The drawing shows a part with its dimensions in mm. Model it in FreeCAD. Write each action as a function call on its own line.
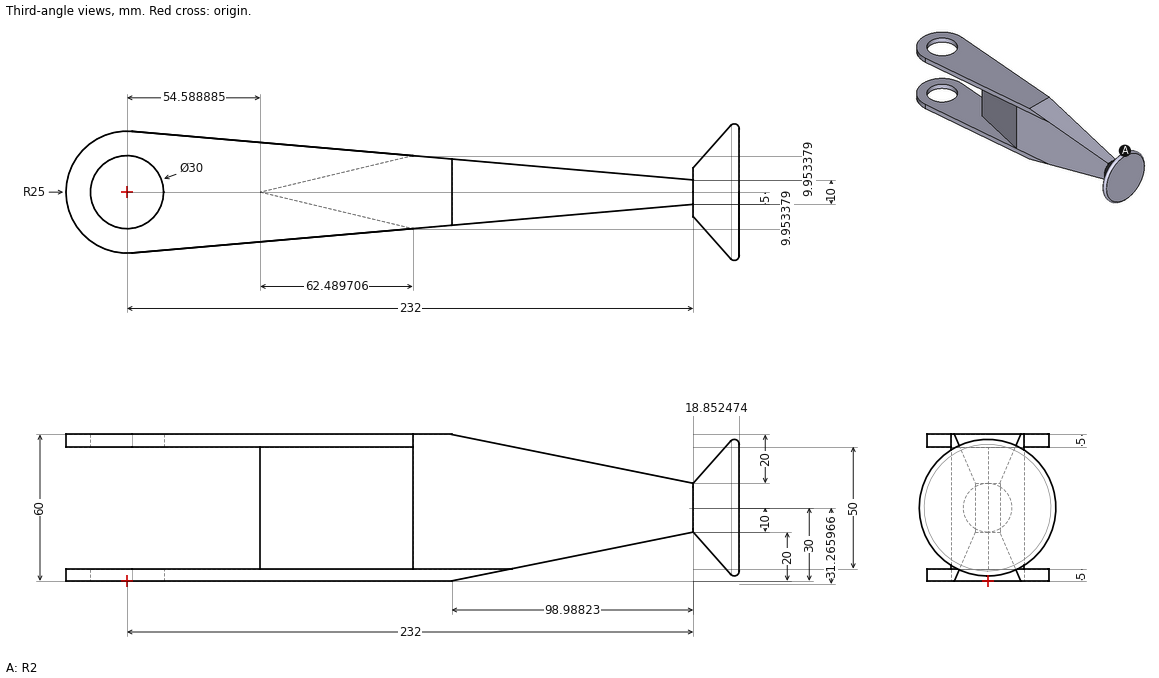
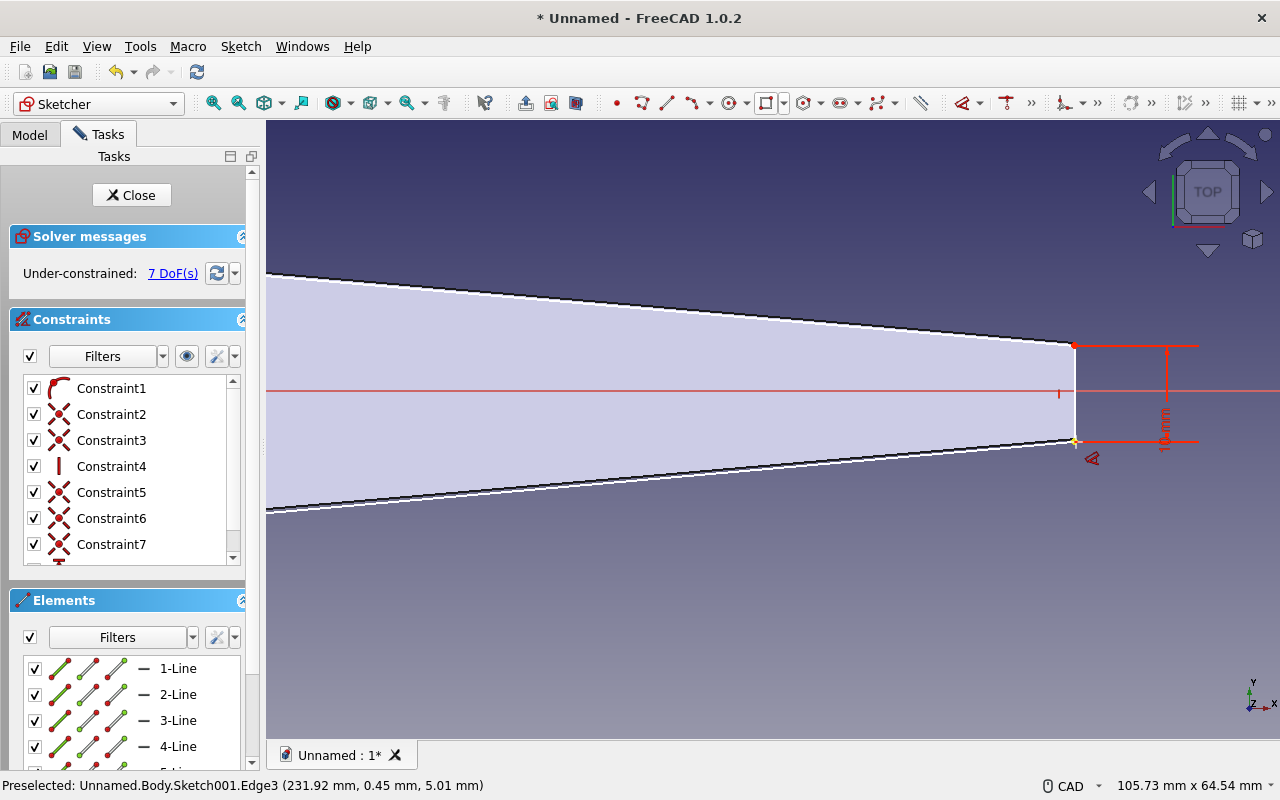
click(1075, 442)
click(1109, 405)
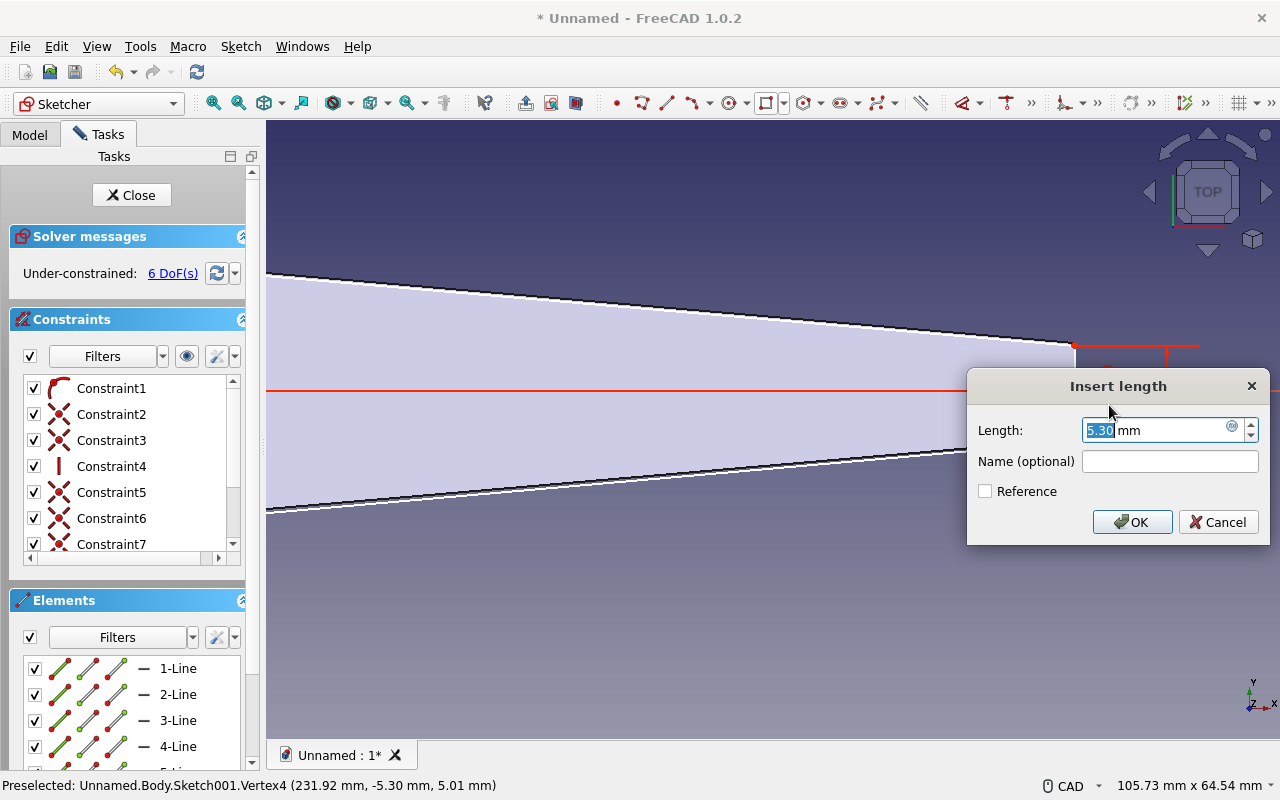
text(5)
key(Return)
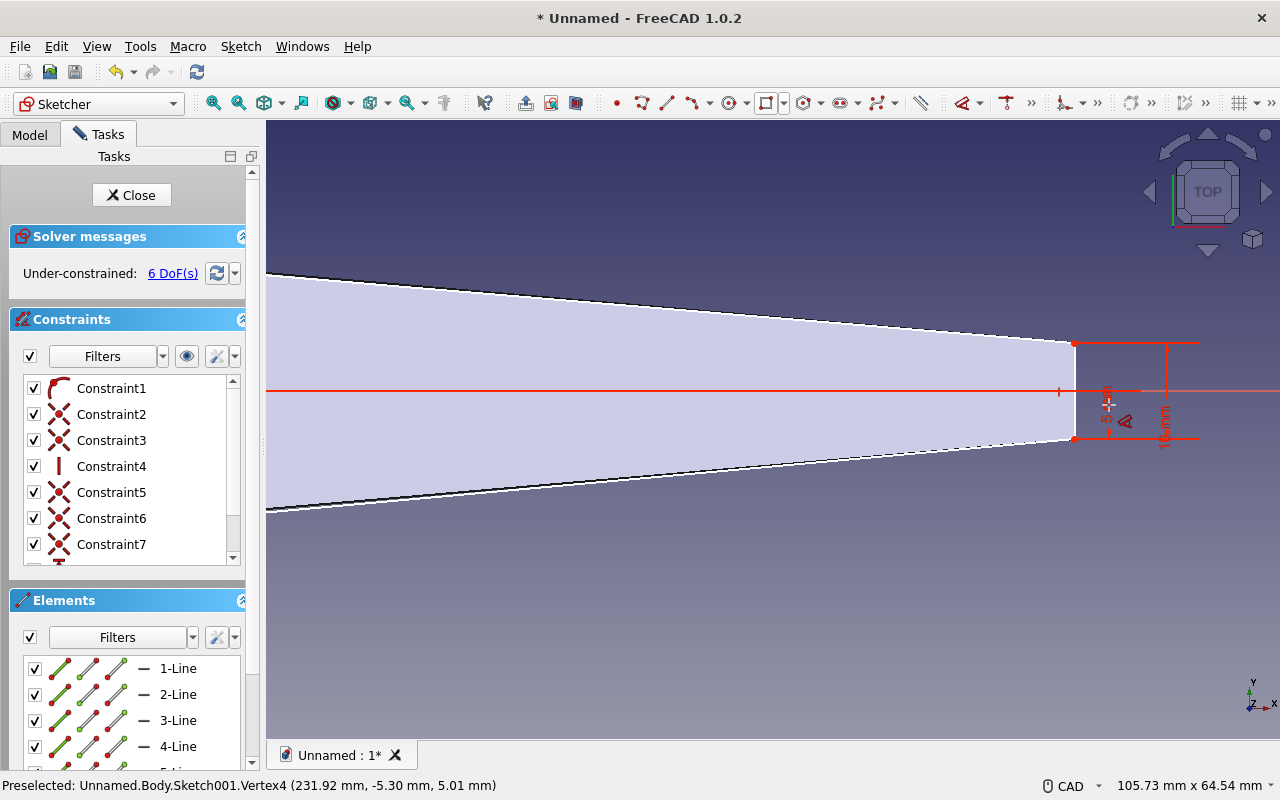
scroll(947, 442, down, 7)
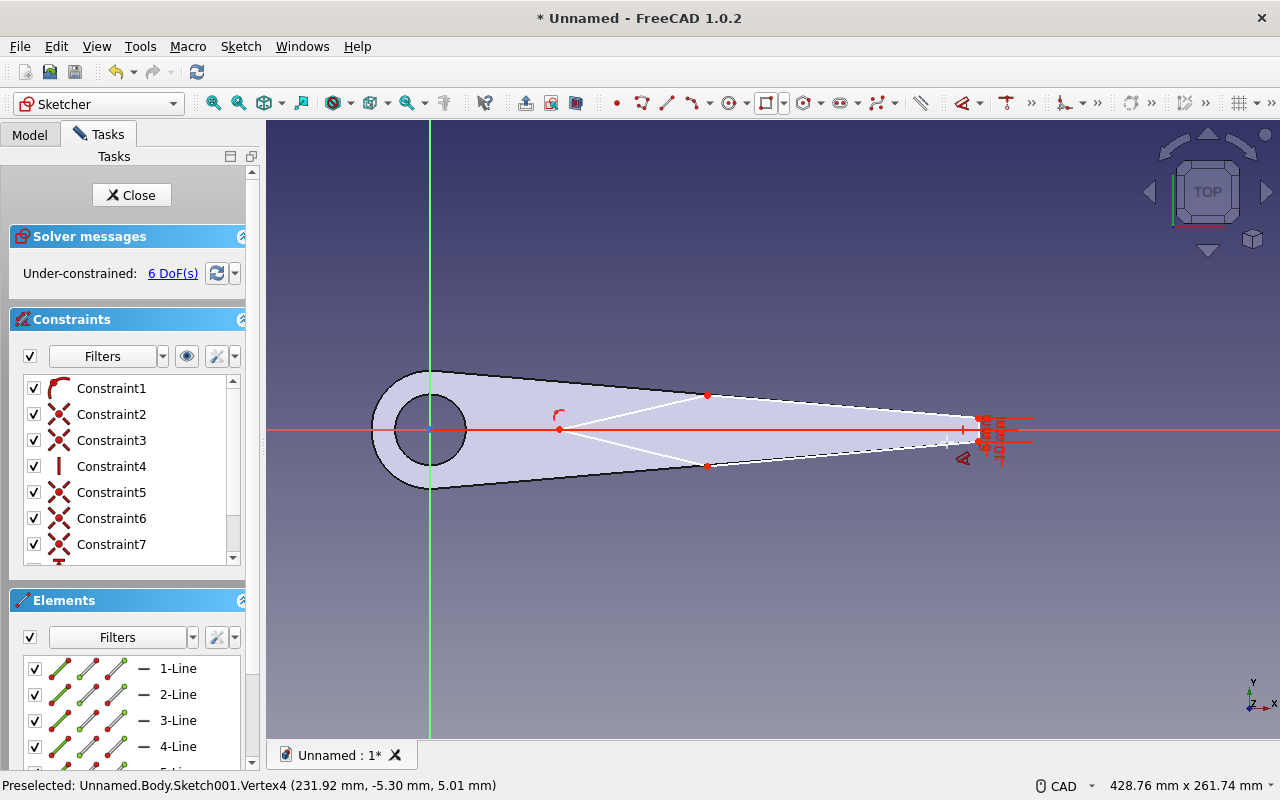
click(979, 442)
click(579, 476)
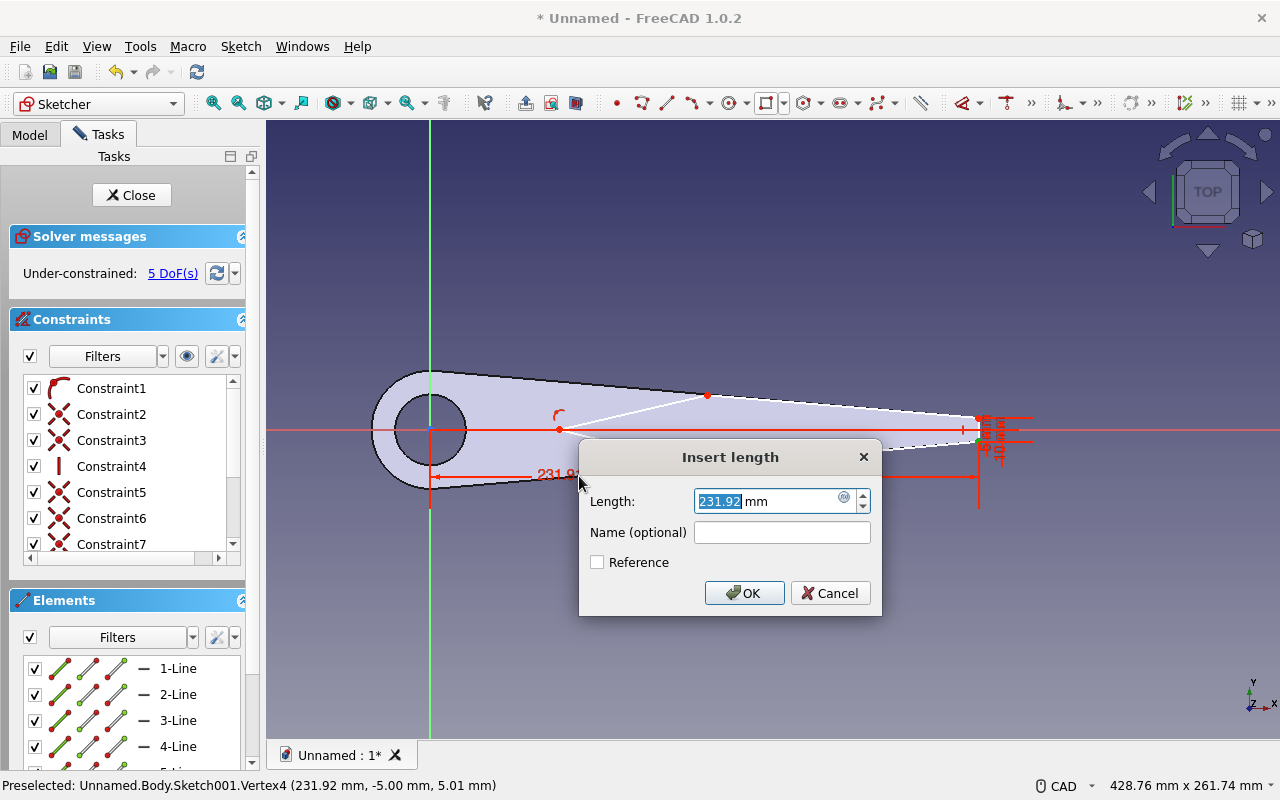
text(232)
key(Return)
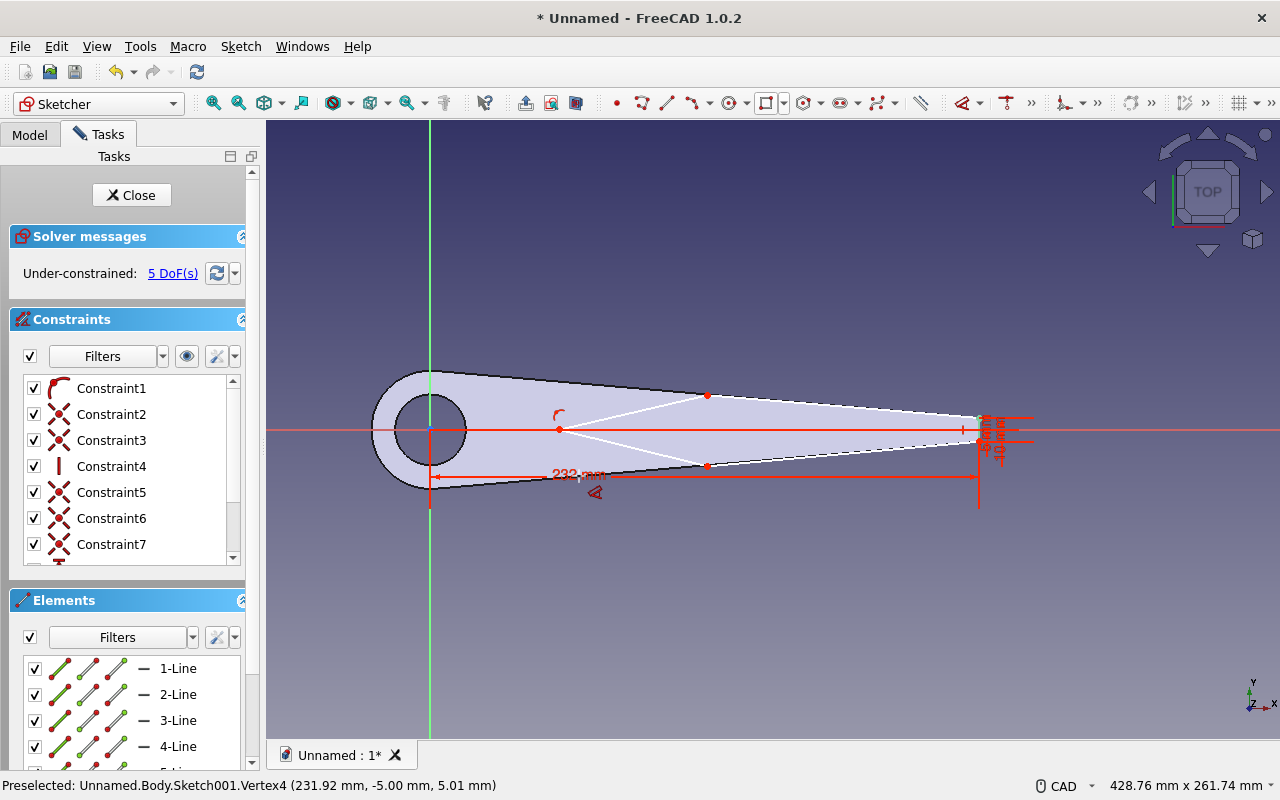
scroll(789, 459, up, 3)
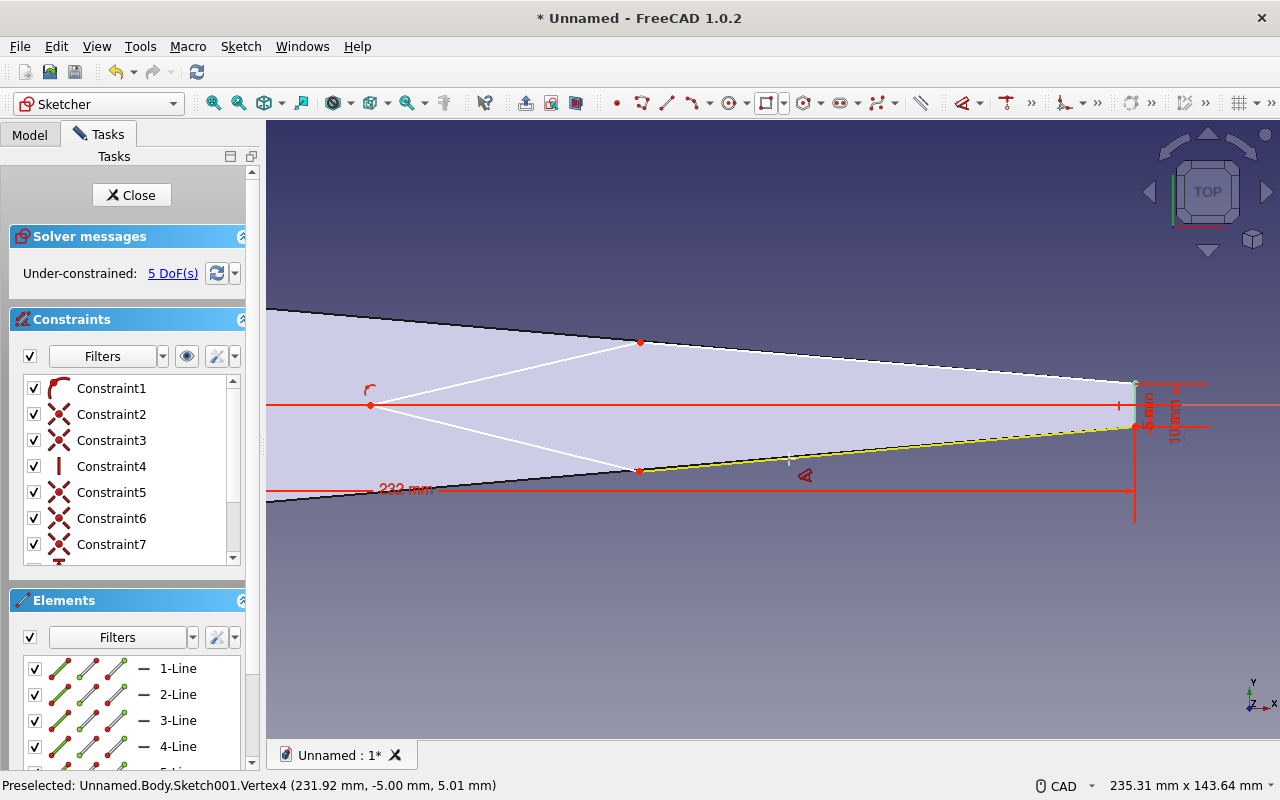
click(788, 458)
click(606, 449)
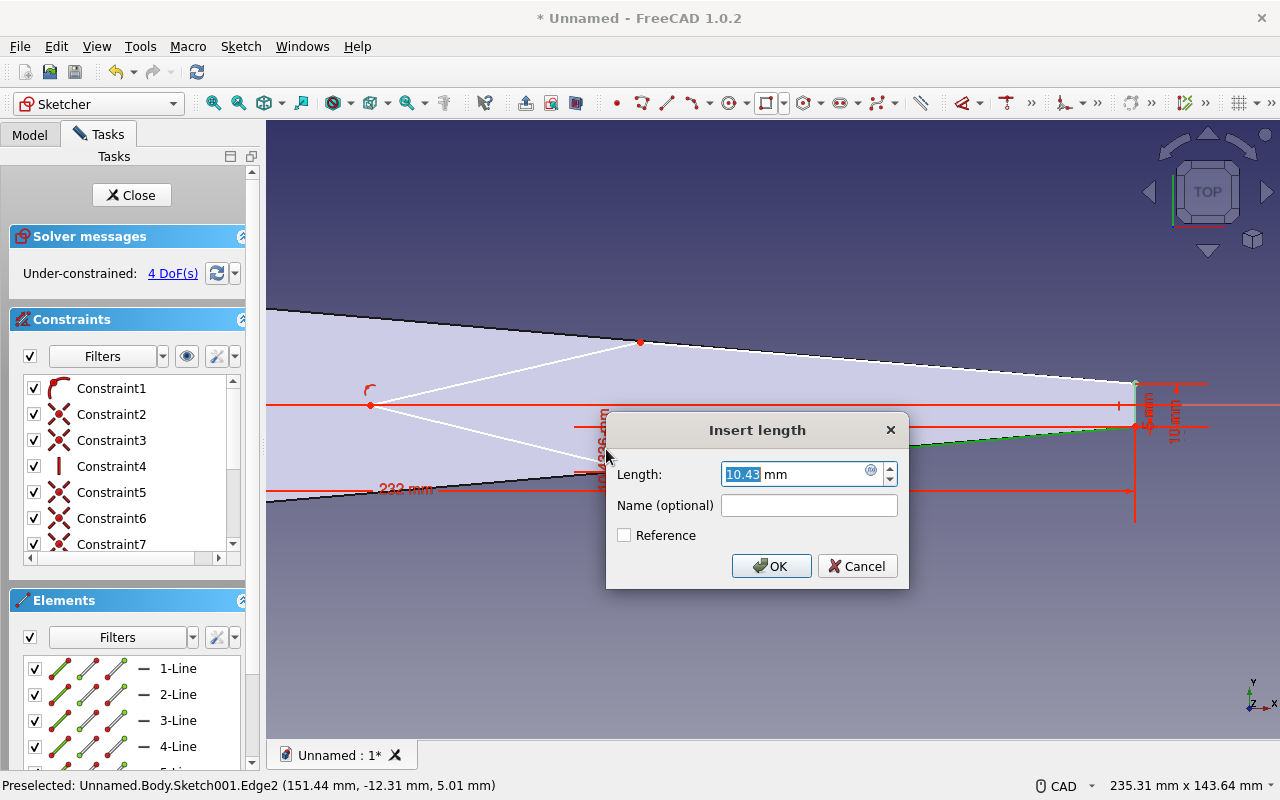
text(9.953379)
key(Return)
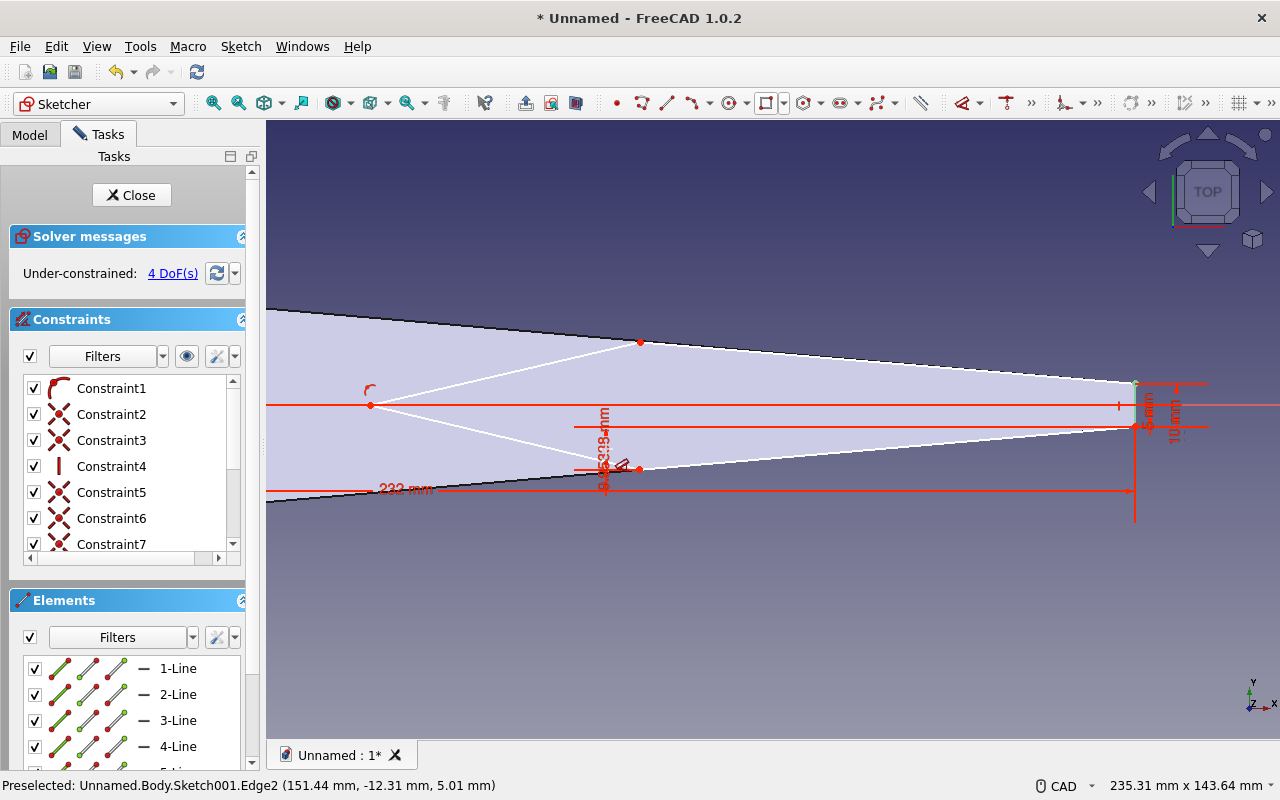
click(987, 371)
click(606, 373)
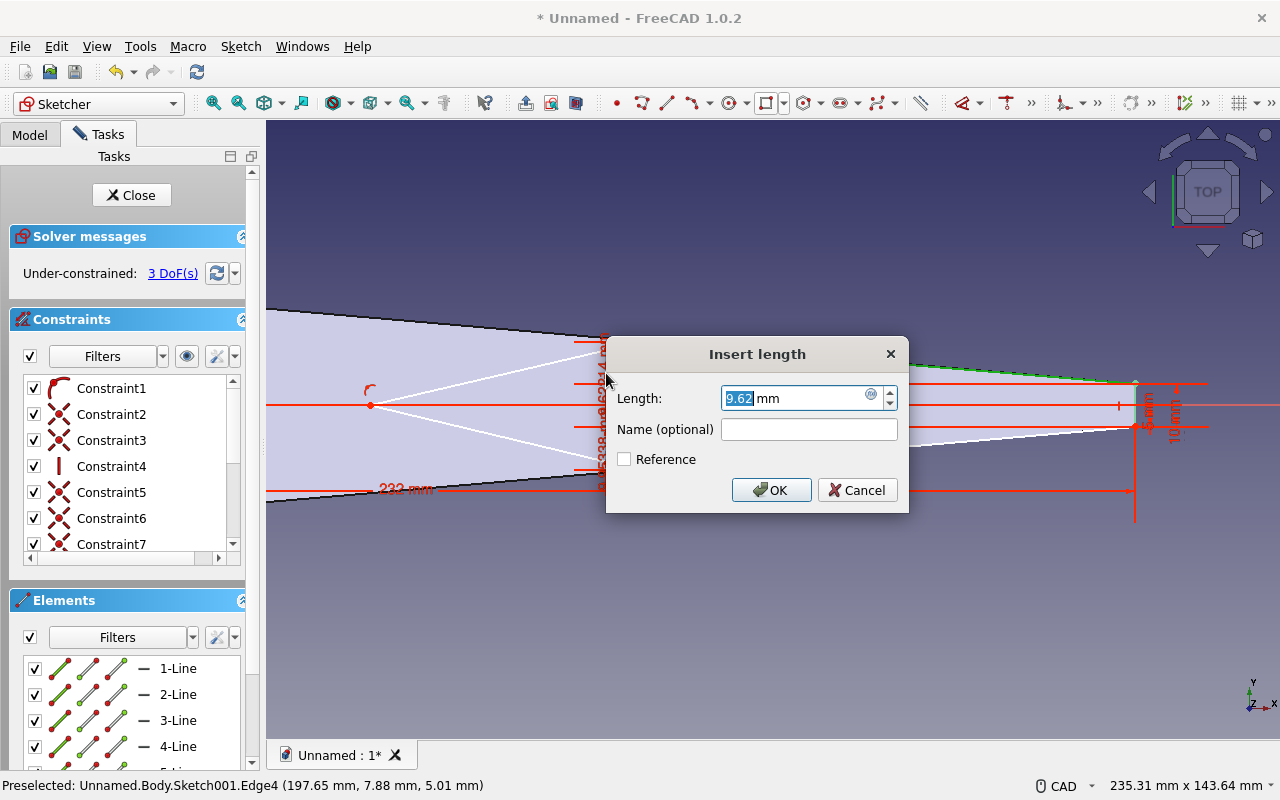
text(9.953379)
key(Return)